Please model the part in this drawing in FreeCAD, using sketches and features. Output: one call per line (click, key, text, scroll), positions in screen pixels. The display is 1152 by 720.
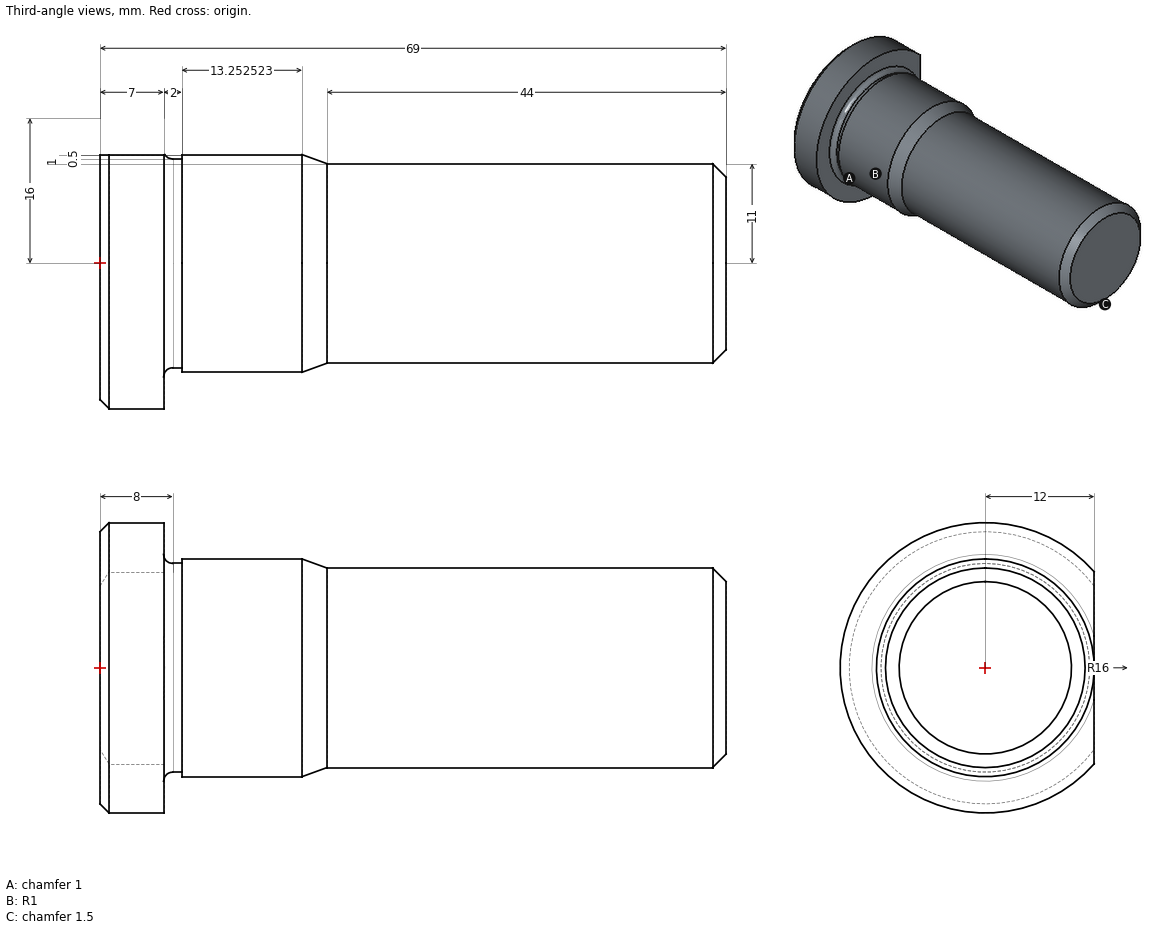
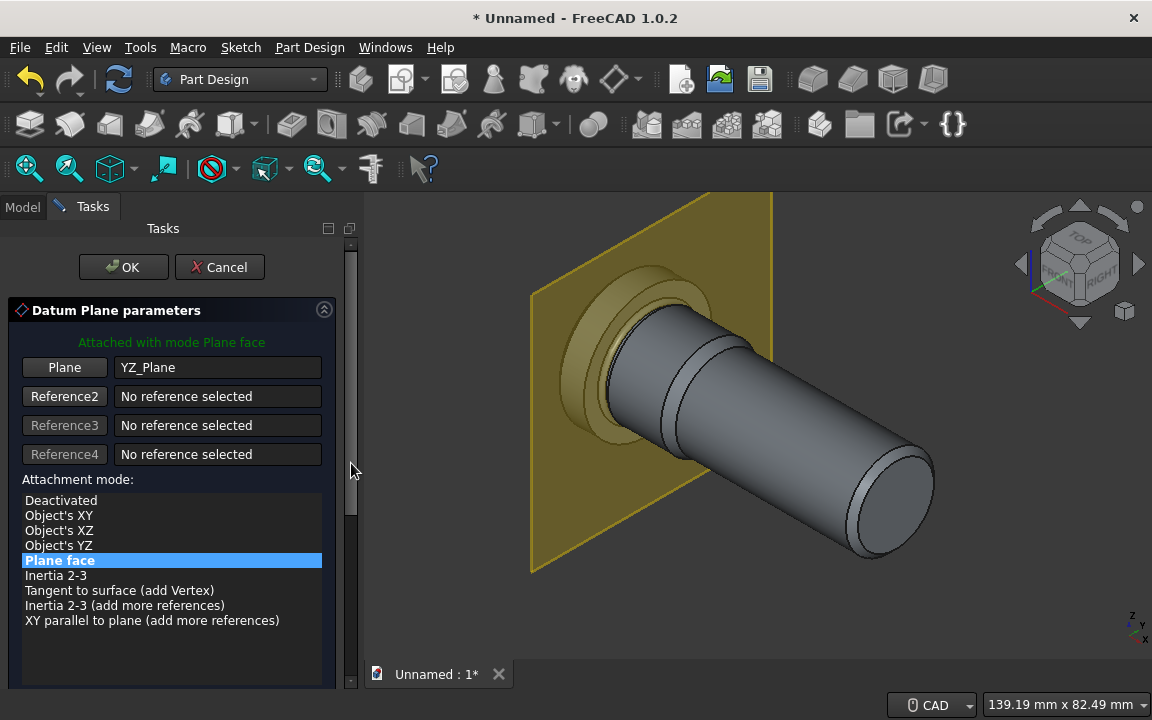
click(124, 267)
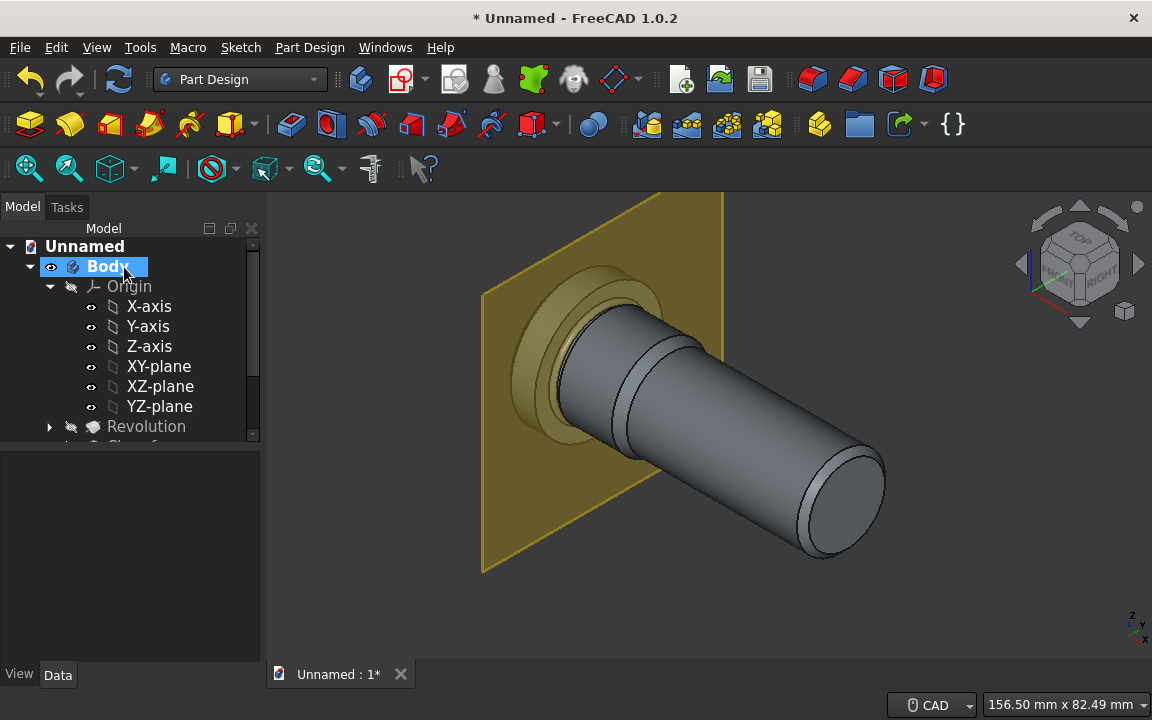
scroll(100, 342, down, 3)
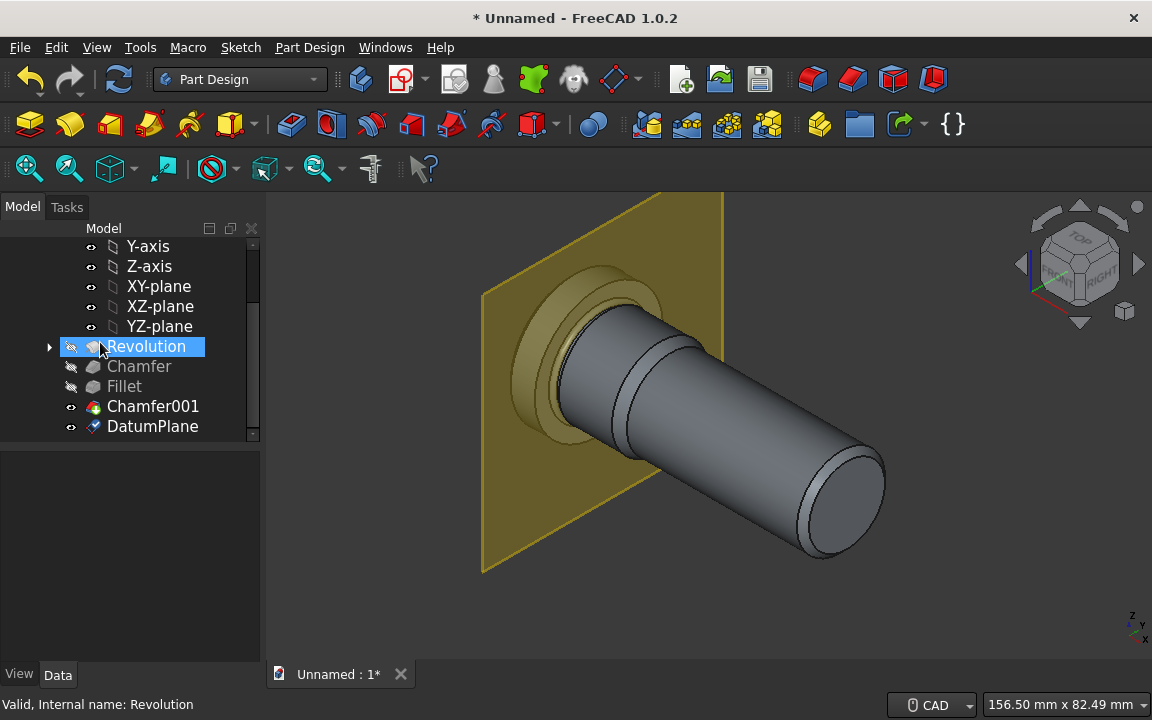
click(116, 427)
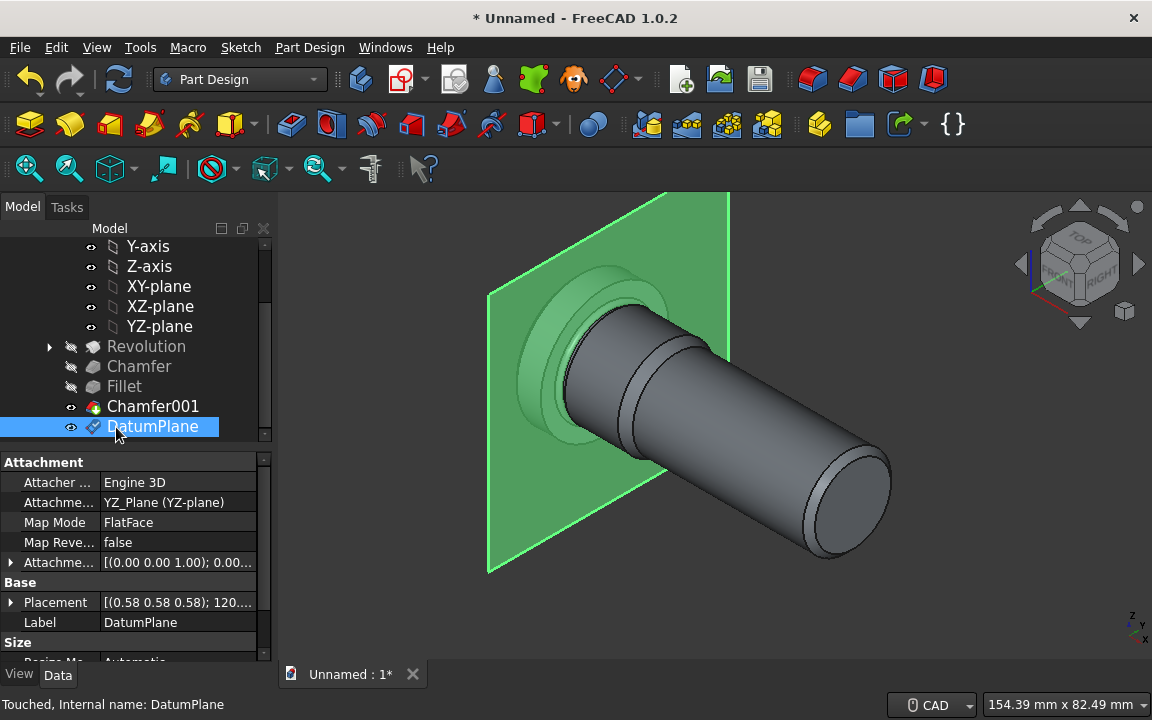
click(402, 80)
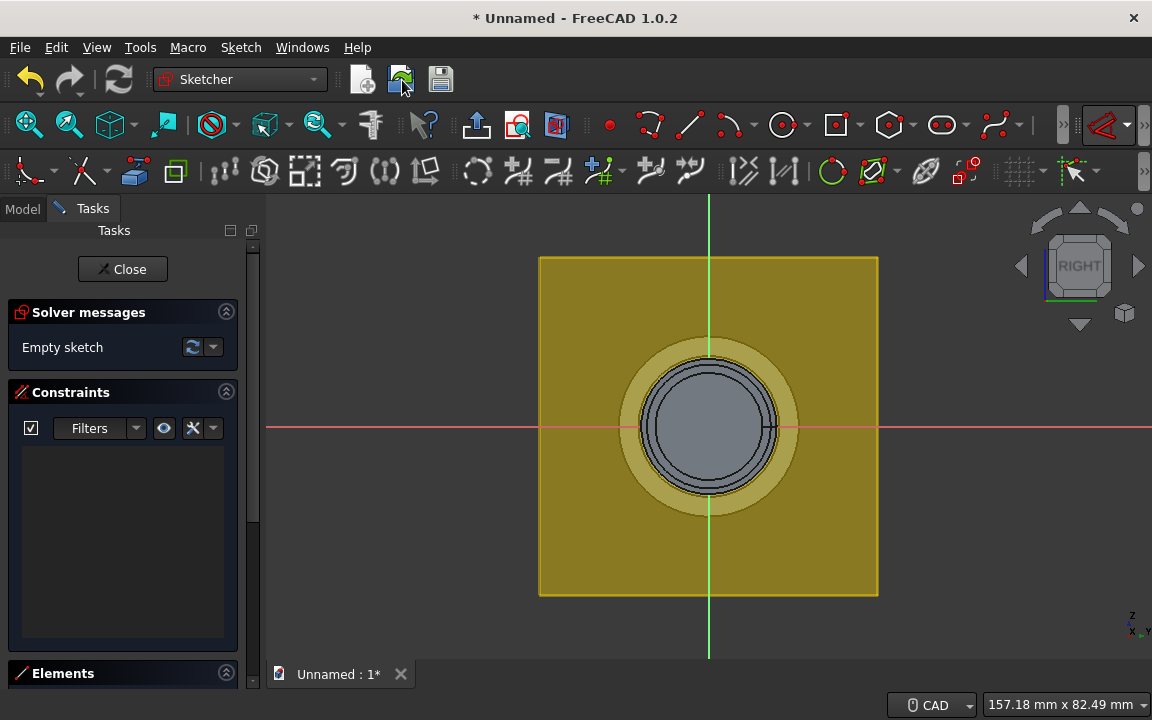
click(558, 126)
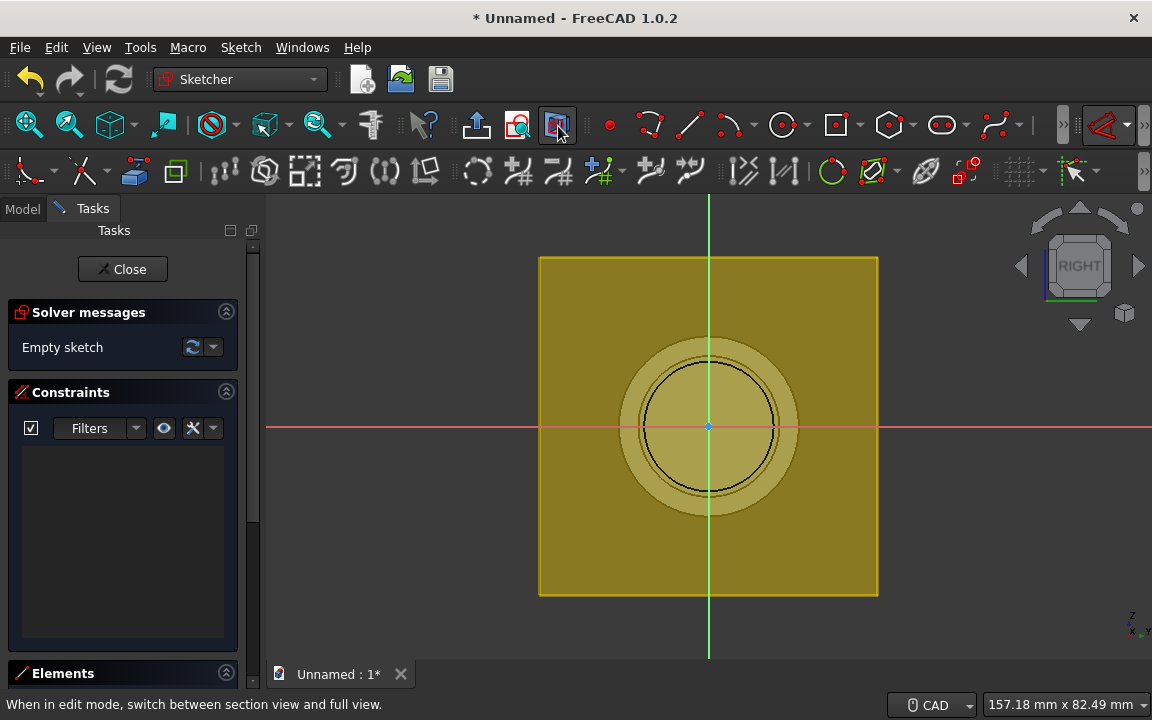
scroll(847, 426, up, 4)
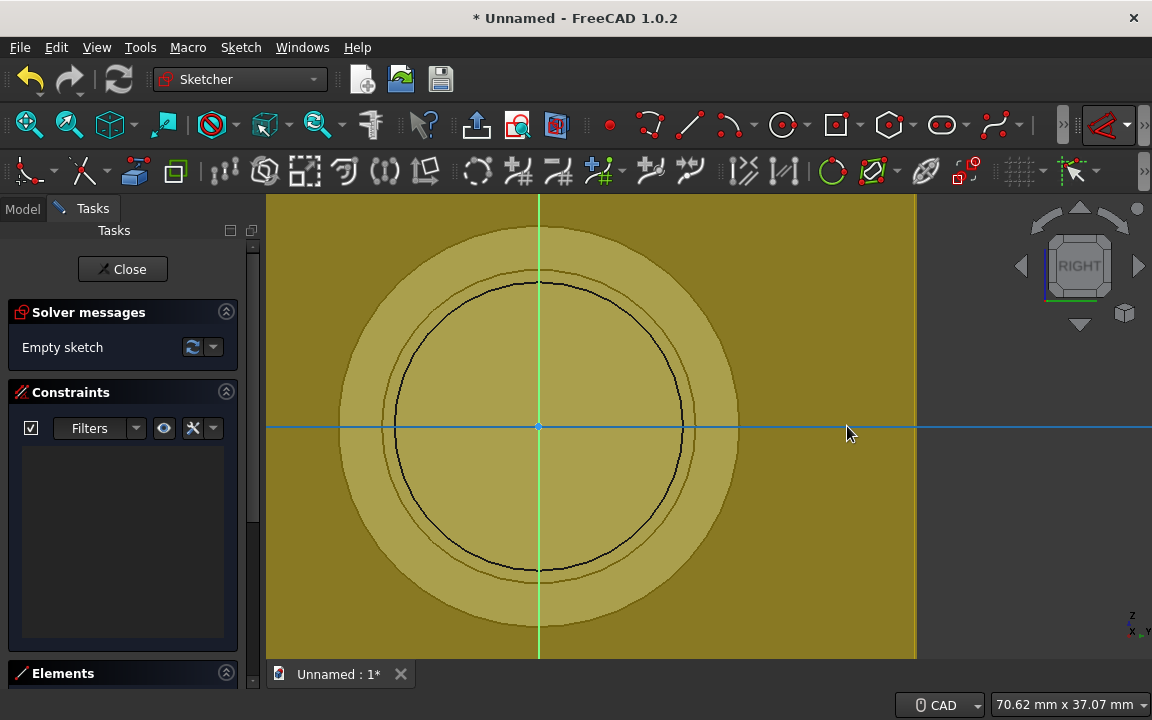
click(690, 126)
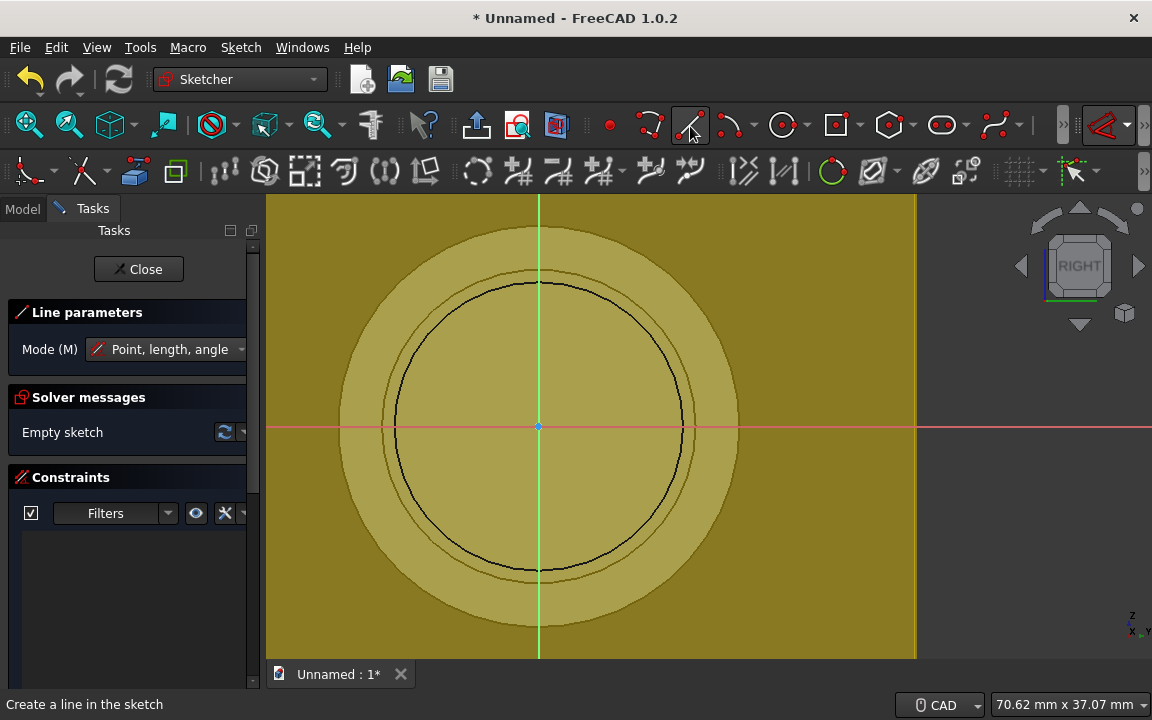
click(689, 294)
click(689, 559)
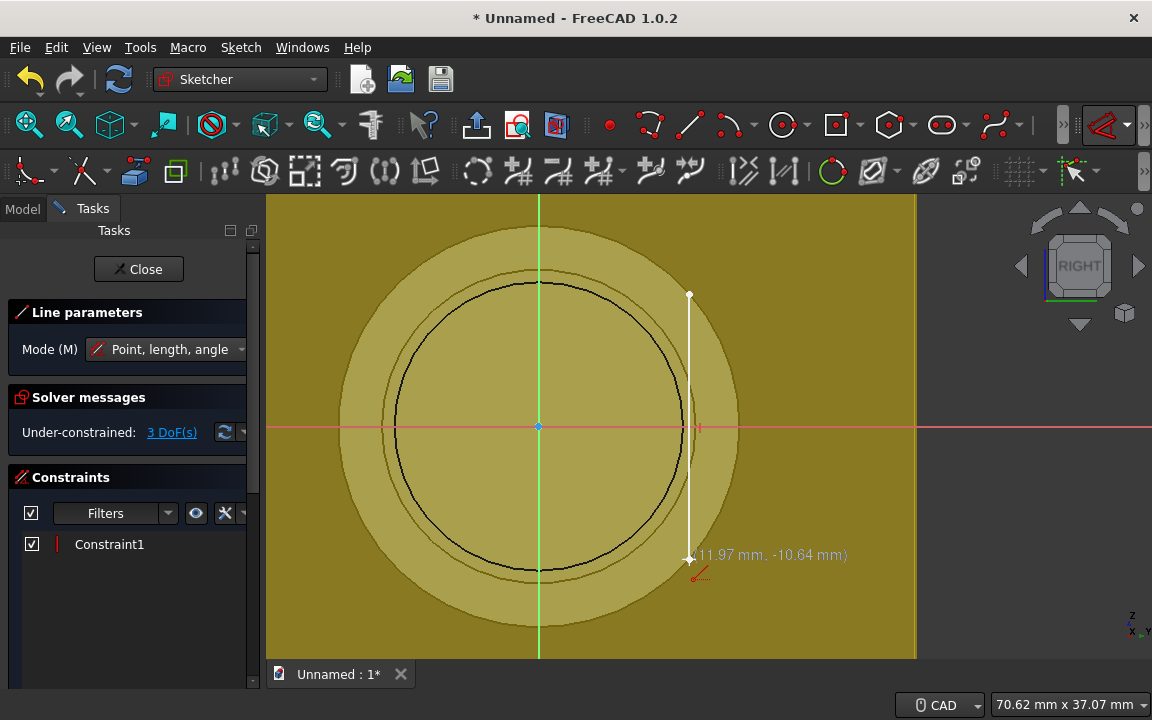
key(g)
key(3)
key(a)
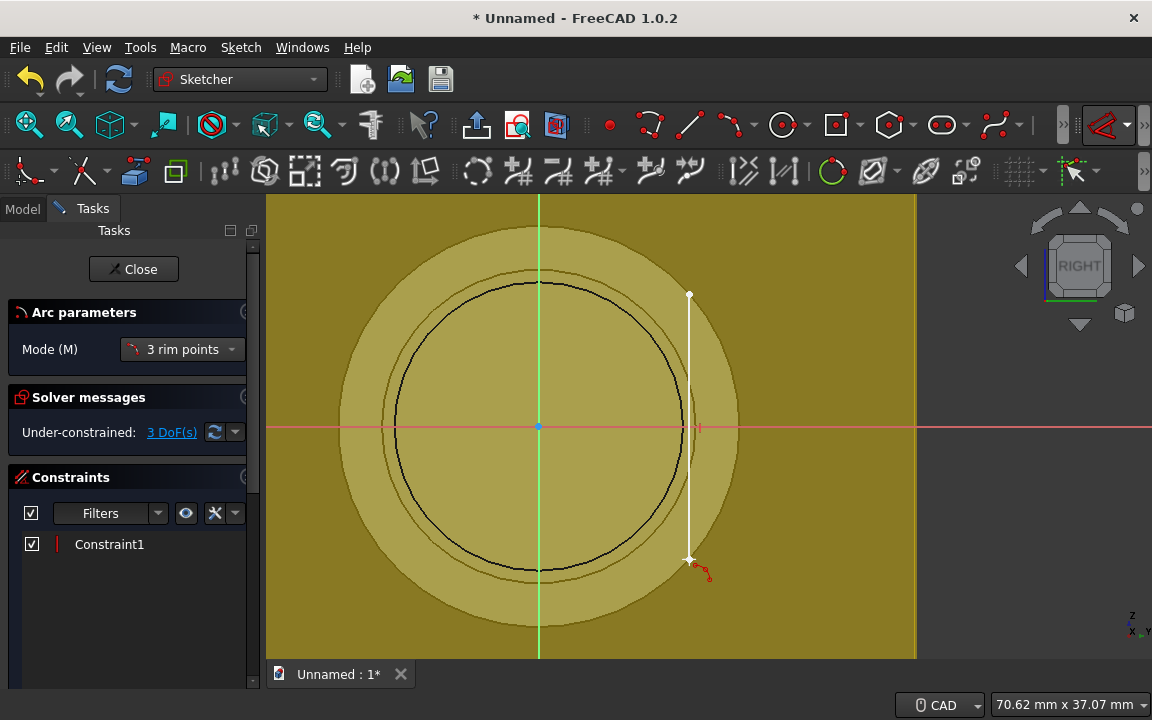
click(689, 560)
click(689, 295)
click(737, 455)
key(Escape)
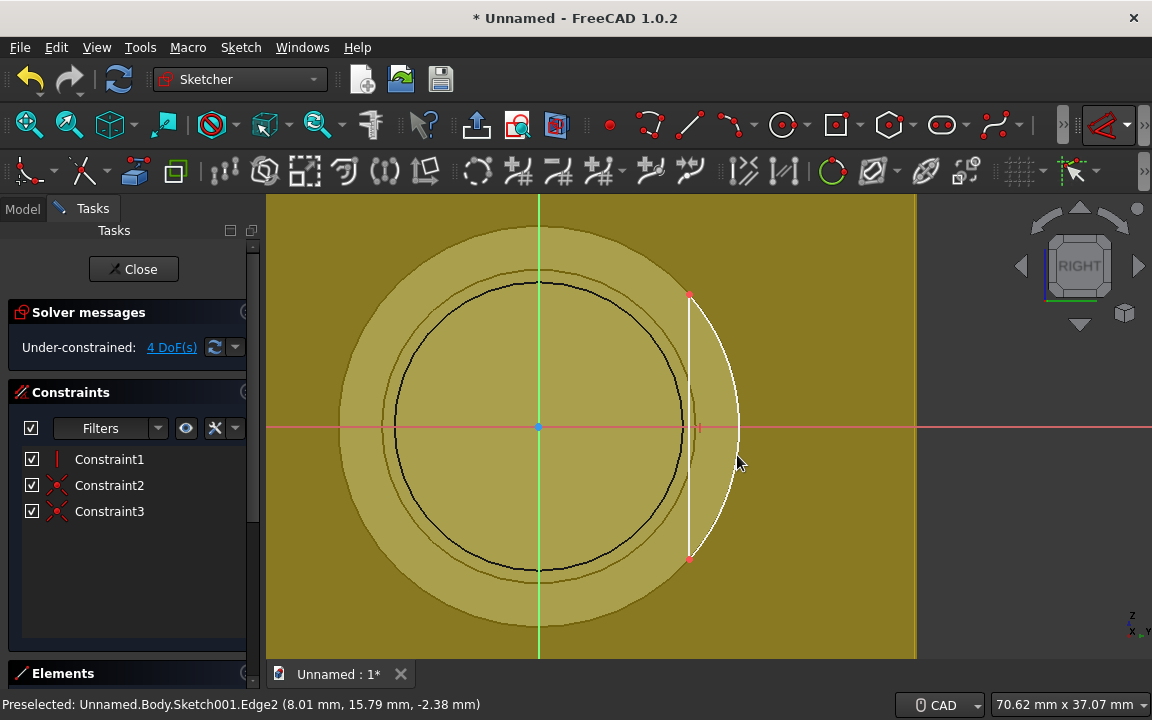
drag(529, 416, 549, 437)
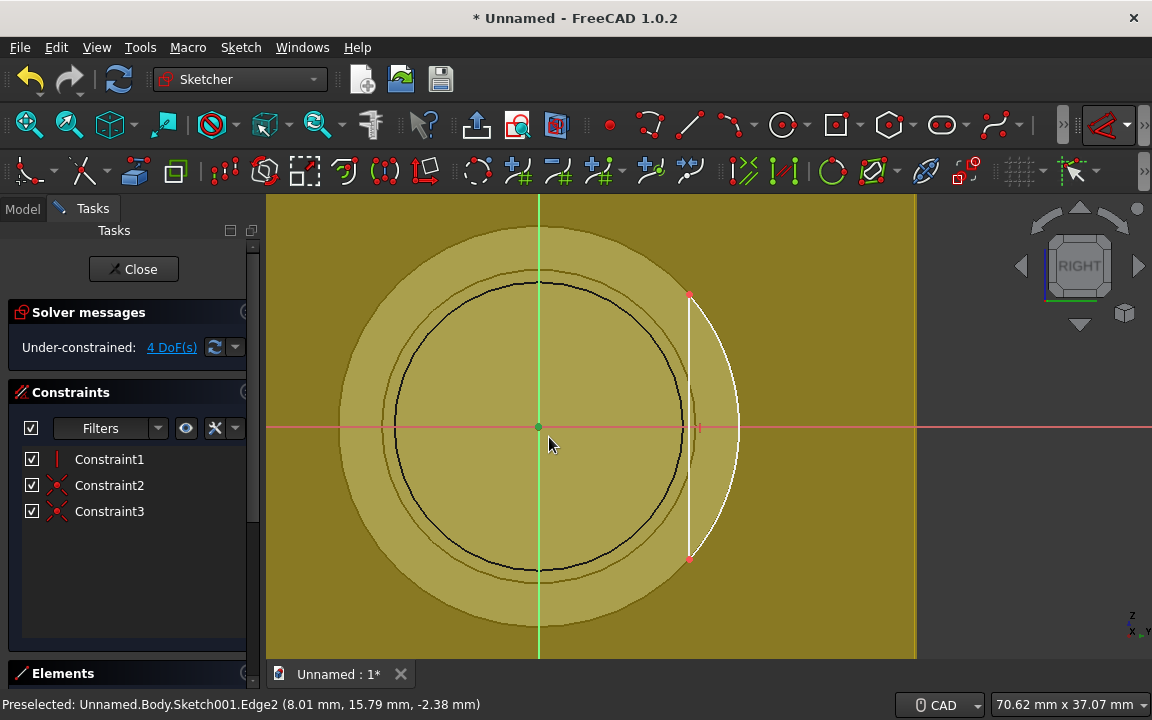
key(c)